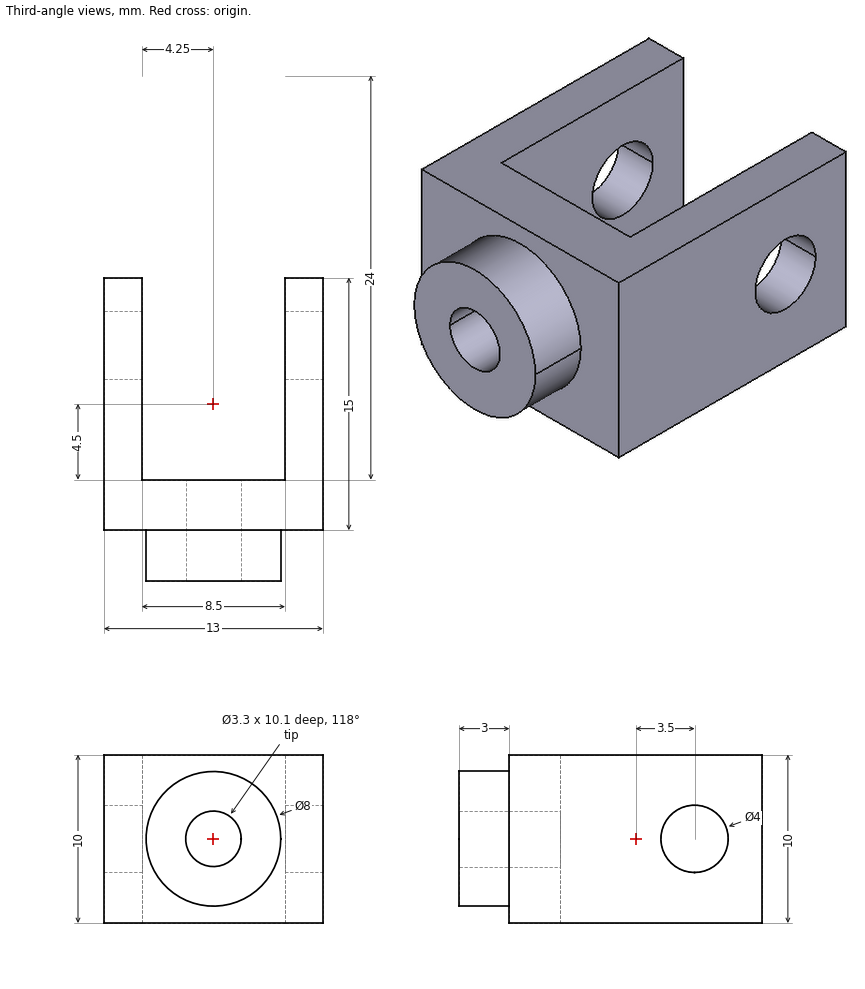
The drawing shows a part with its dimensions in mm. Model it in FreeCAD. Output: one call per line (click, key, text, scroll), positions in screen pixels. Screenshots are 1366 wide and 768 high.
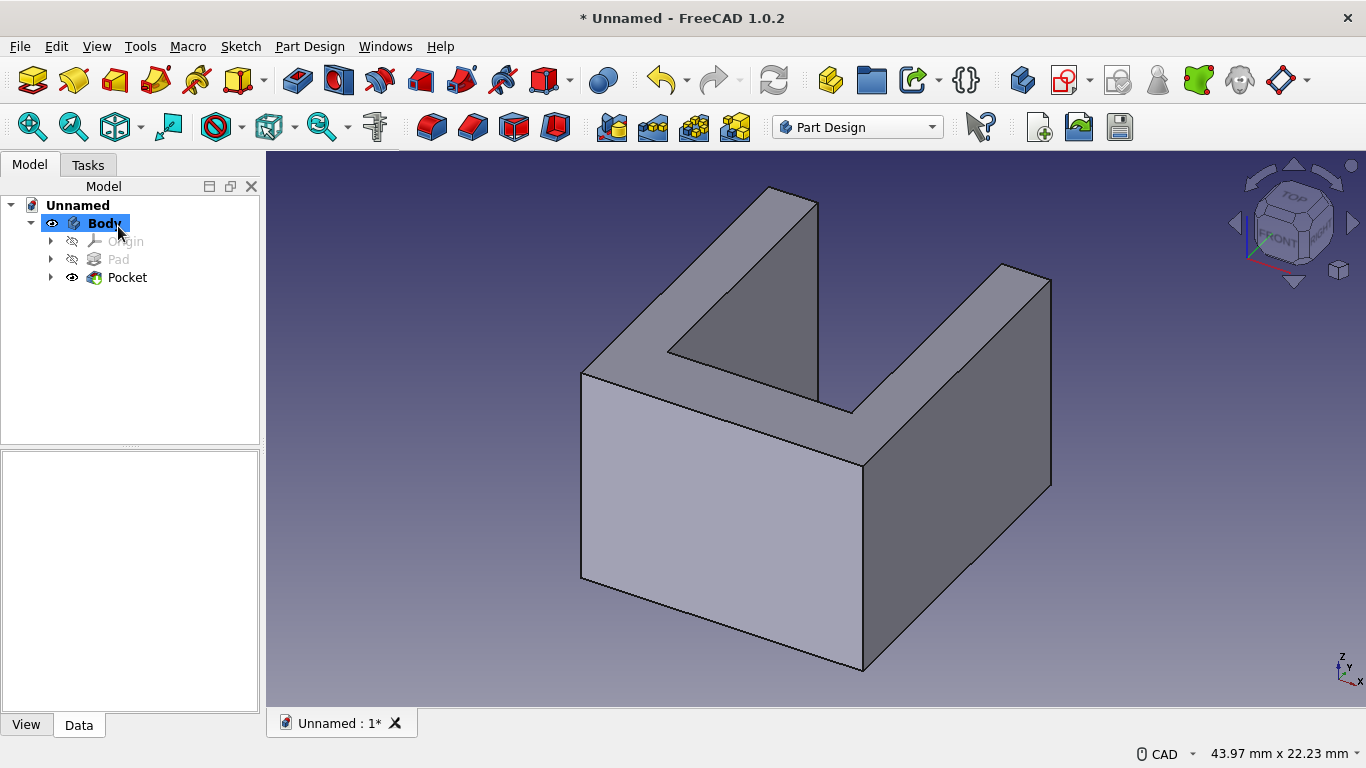
click(984, 448)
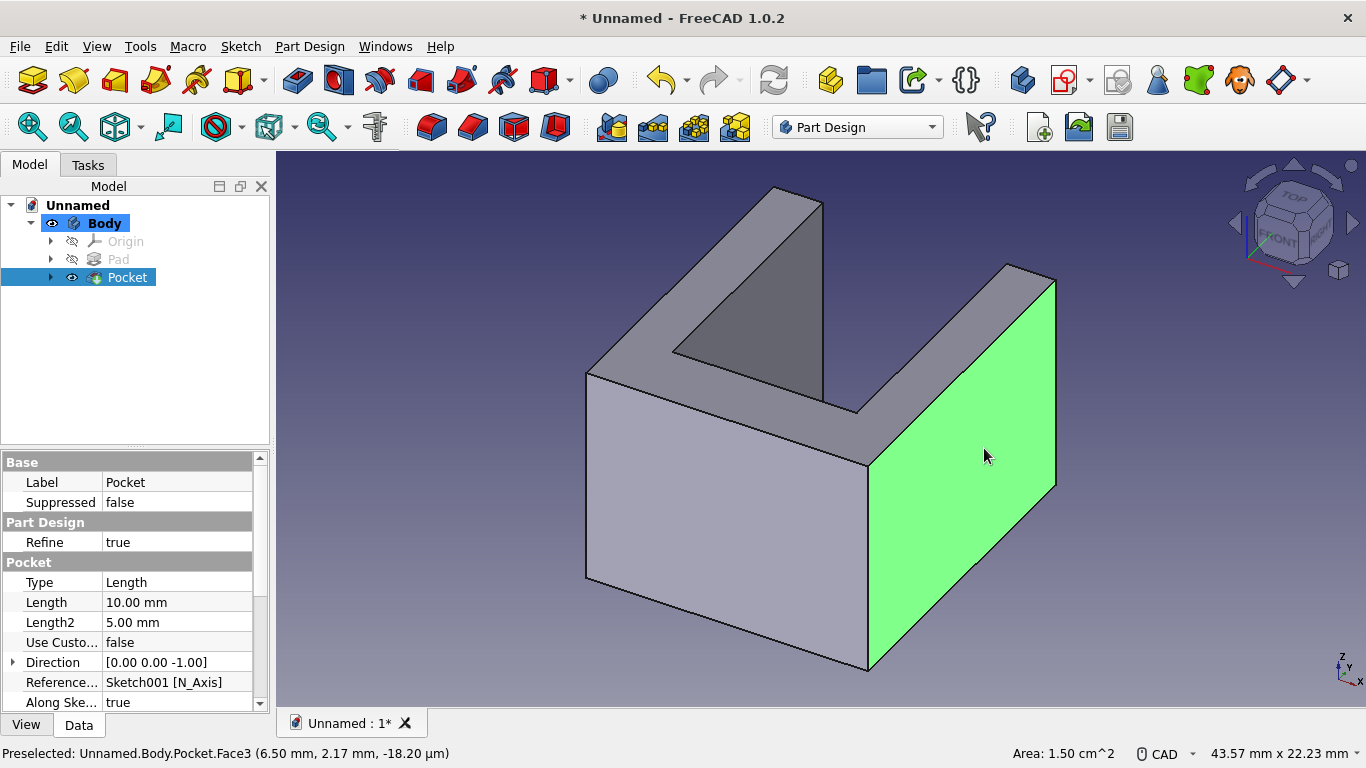
click(1064, 80)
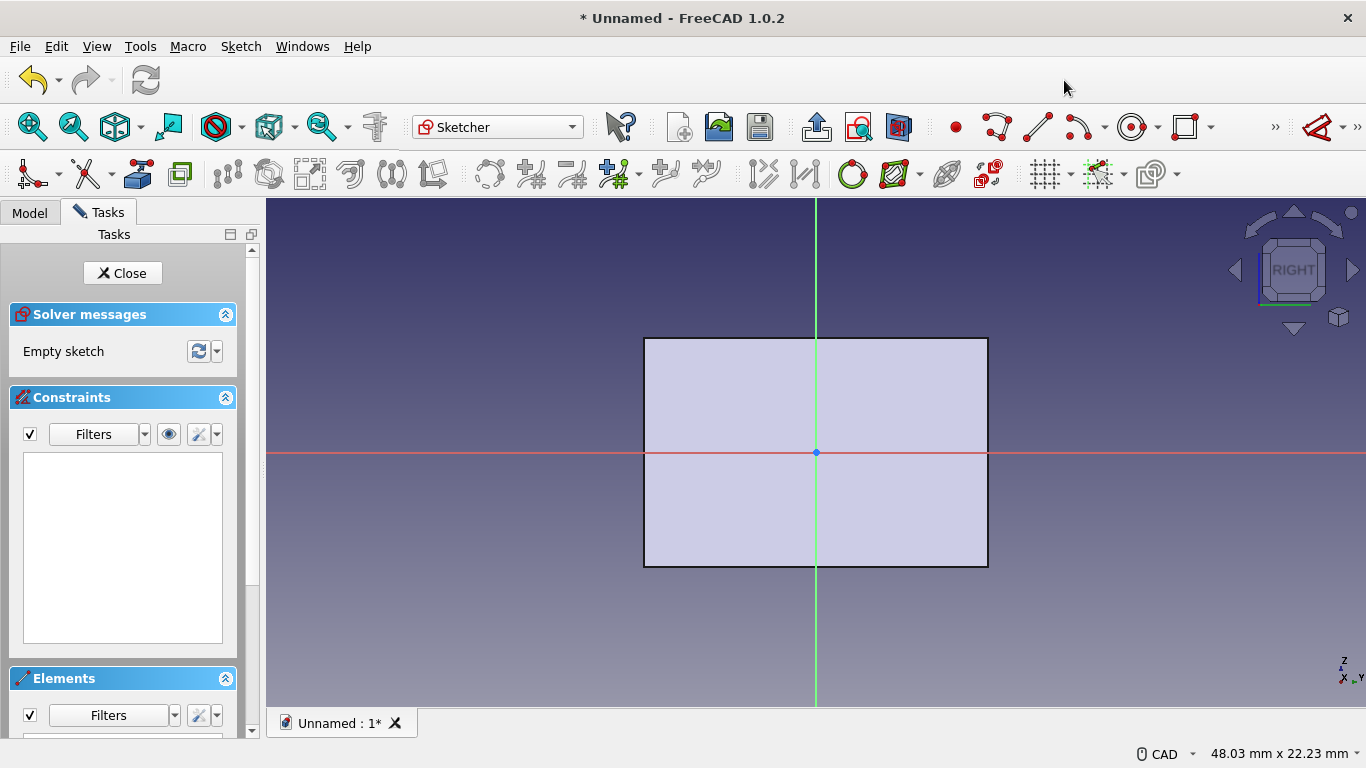
scroll(936, 452, up, 6)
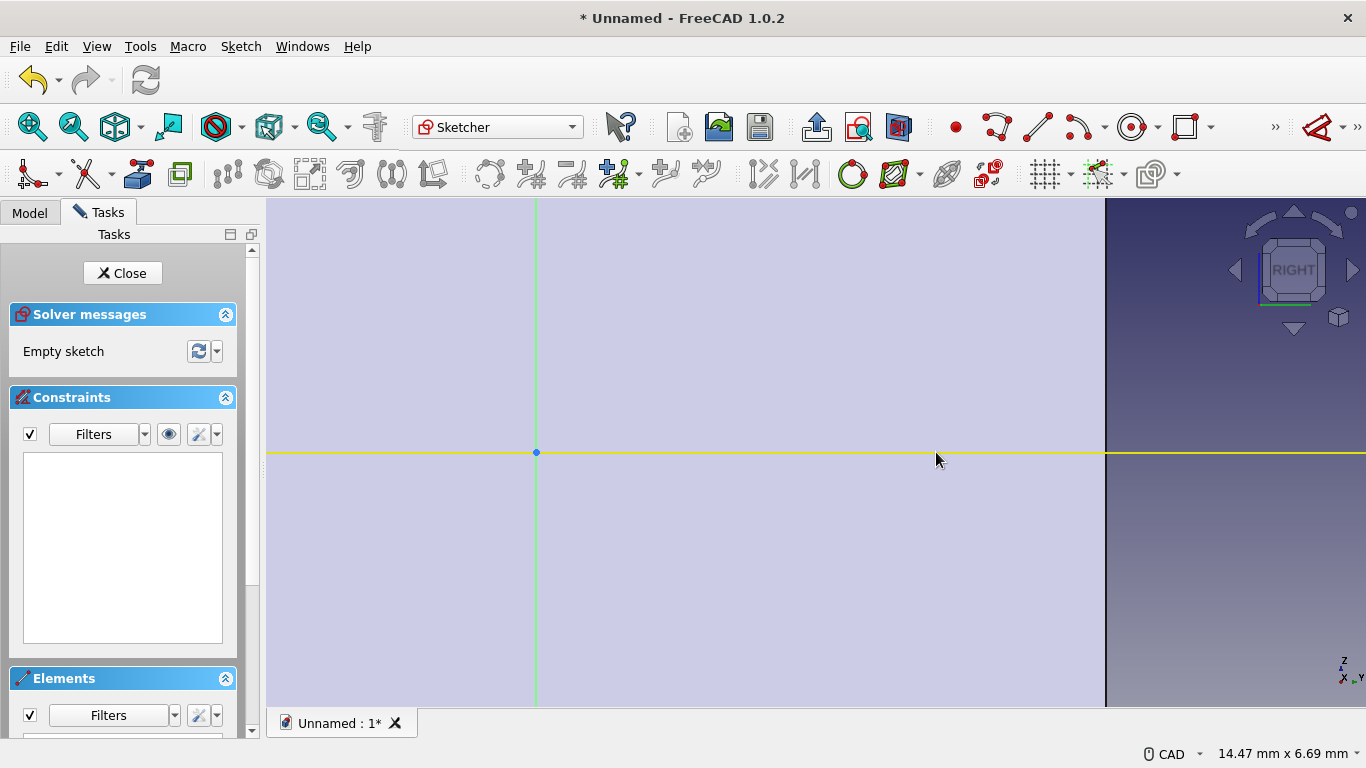
click(1132, 128)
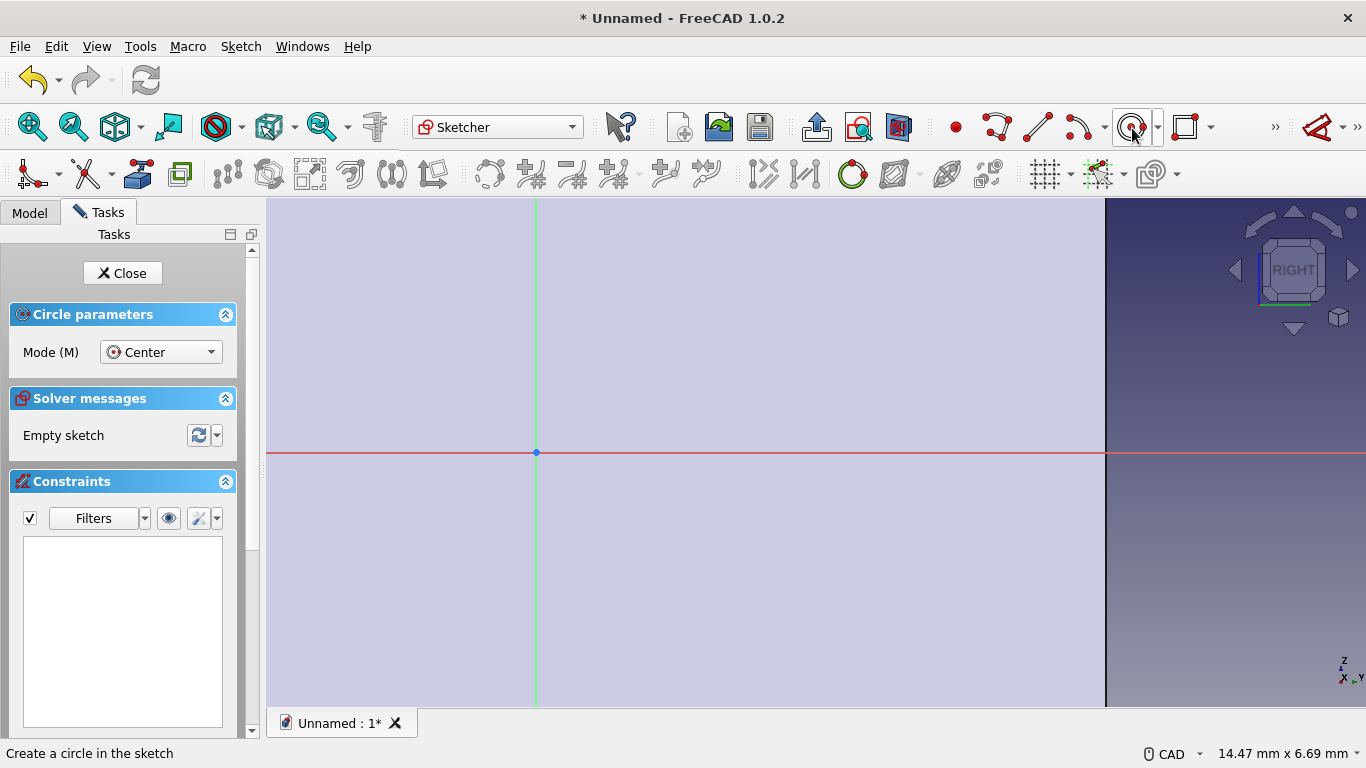
click(802, 452)
move(910, 345)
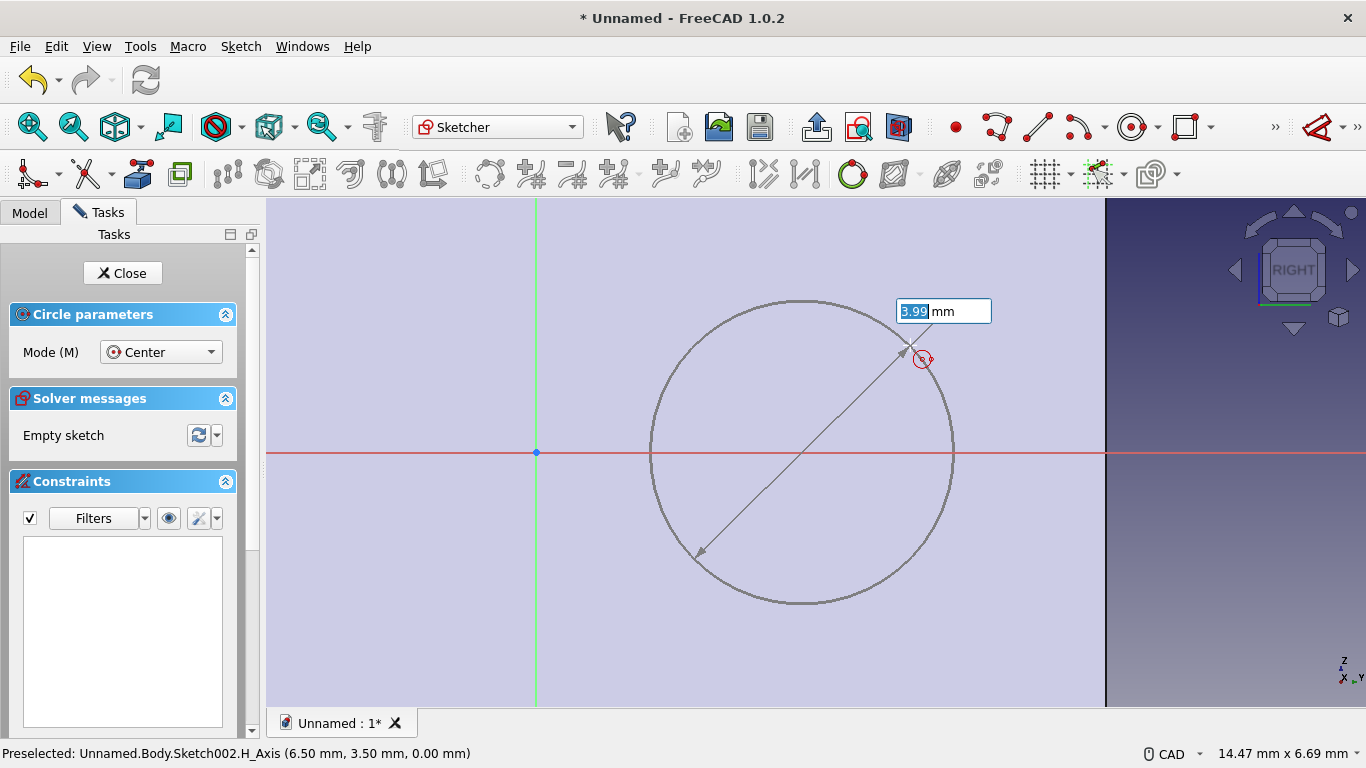
text(4)
key(Return)
key(Escape)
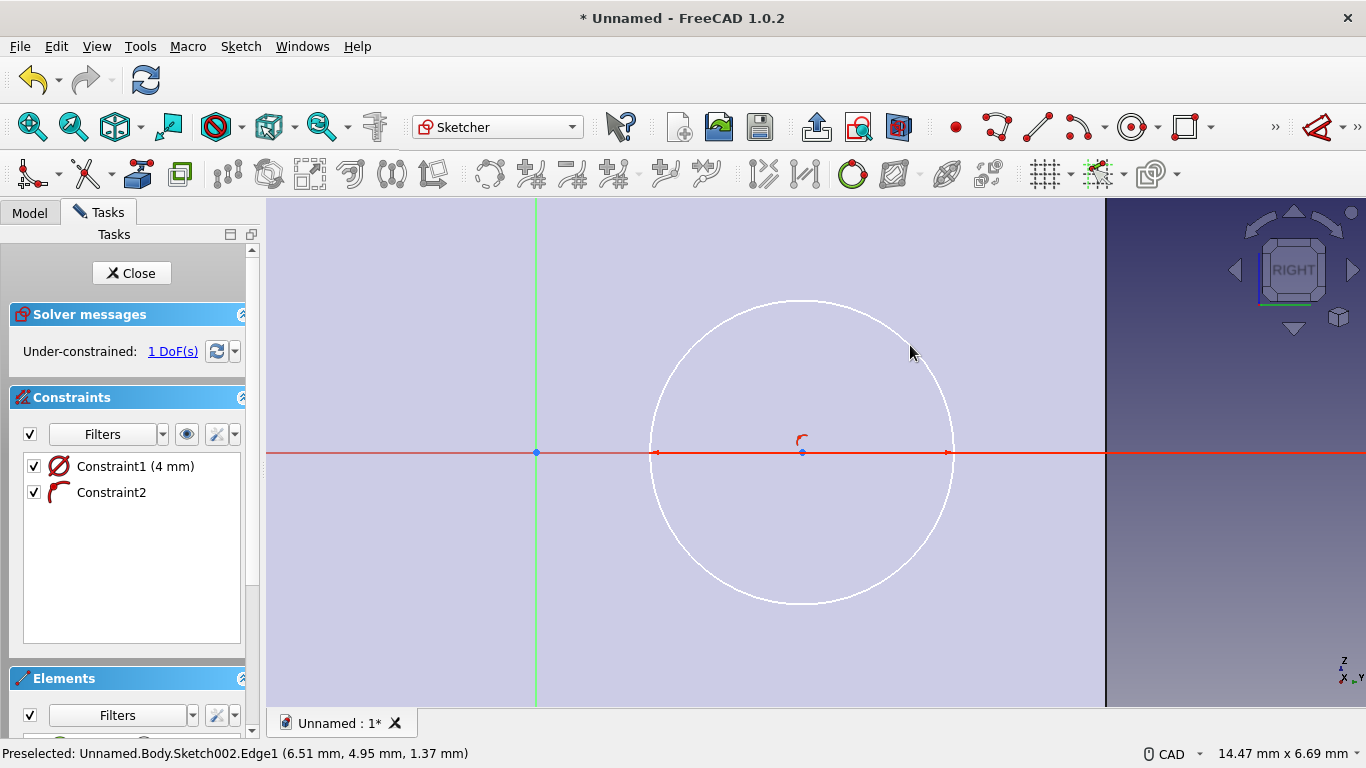
click(802, 452)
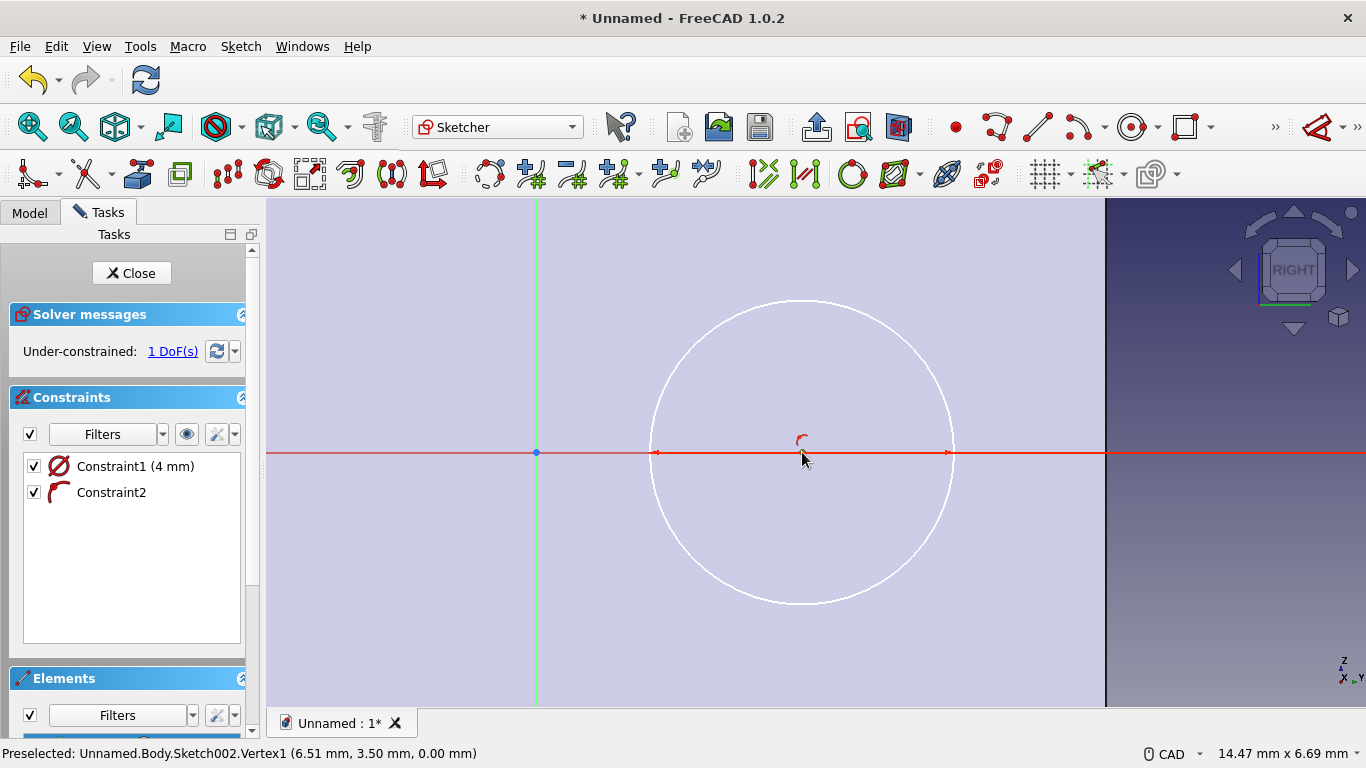
key(l)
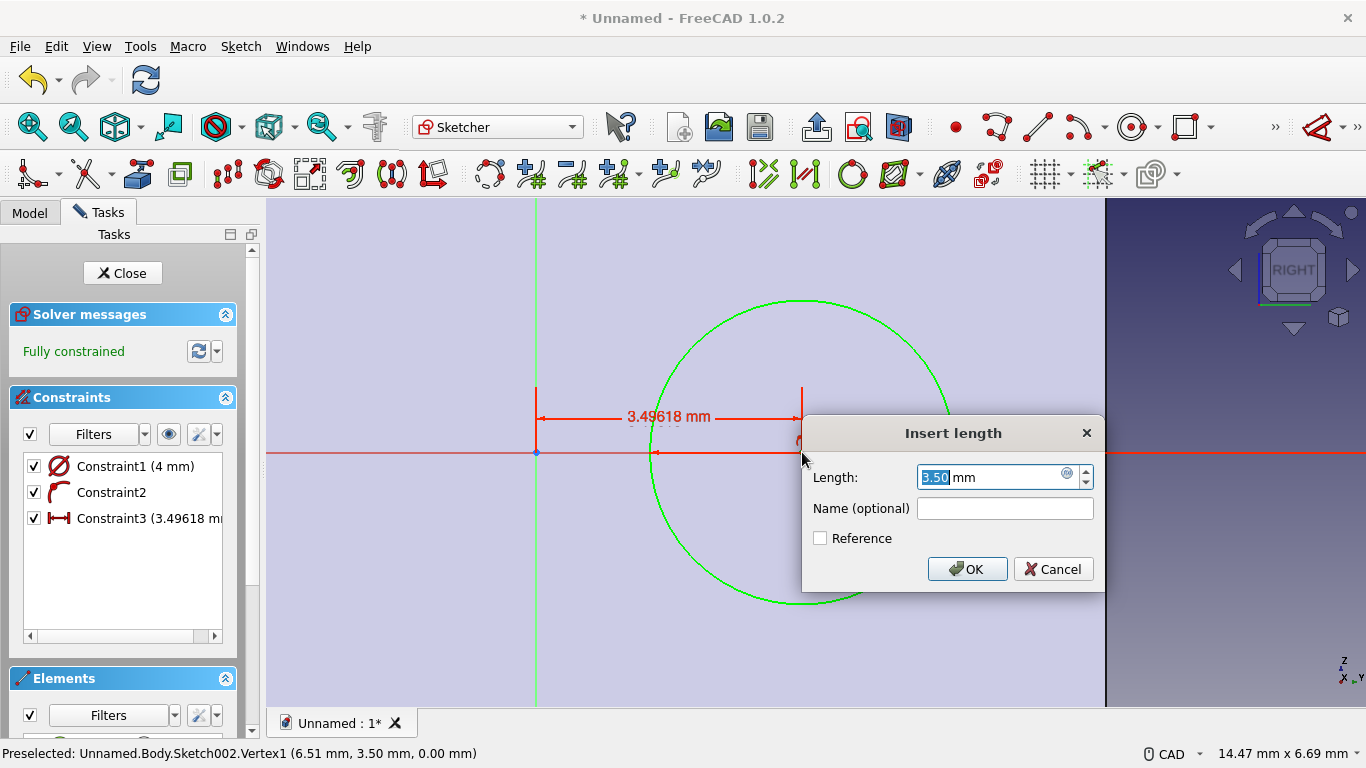
text(3.5)
key(Return)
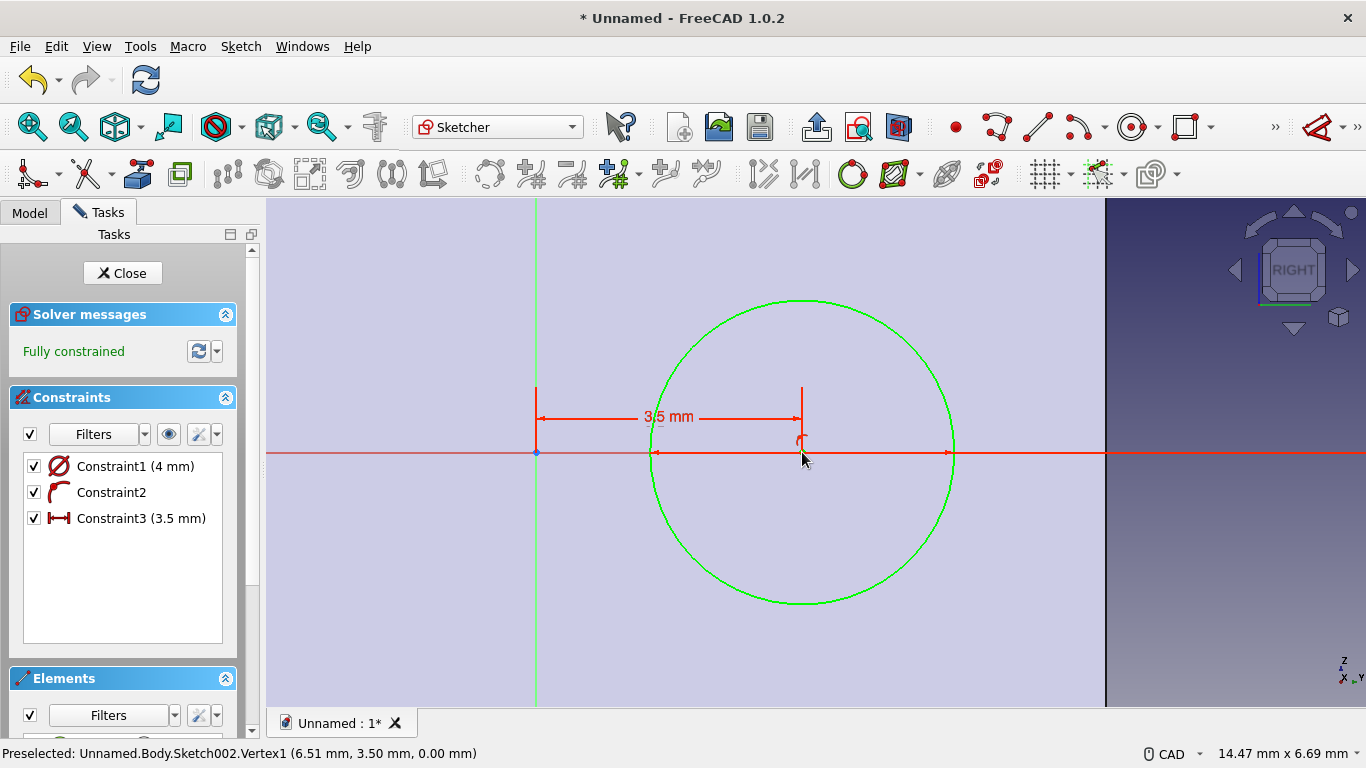
click(123, 273)